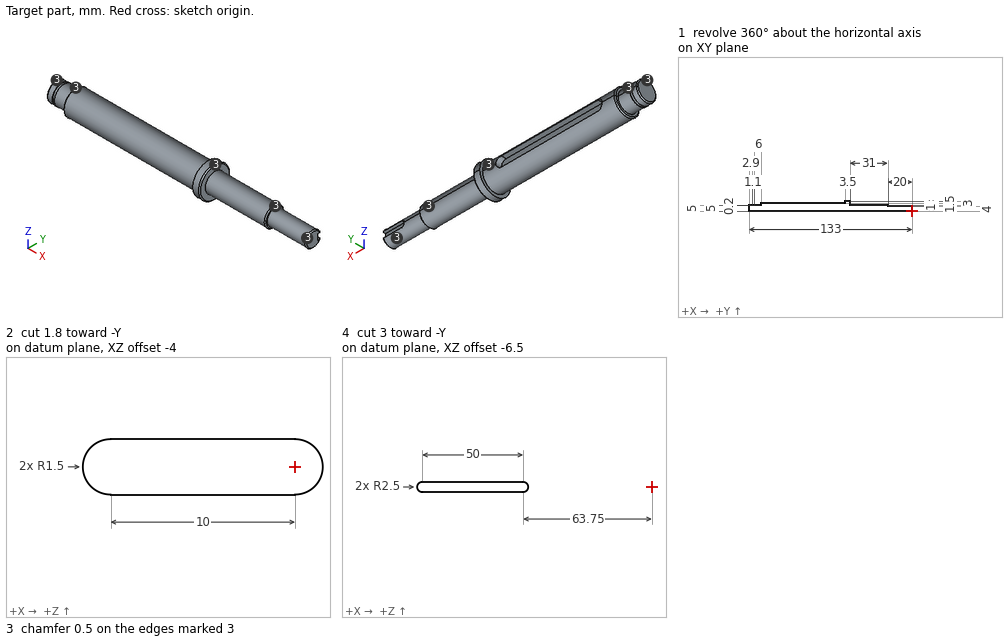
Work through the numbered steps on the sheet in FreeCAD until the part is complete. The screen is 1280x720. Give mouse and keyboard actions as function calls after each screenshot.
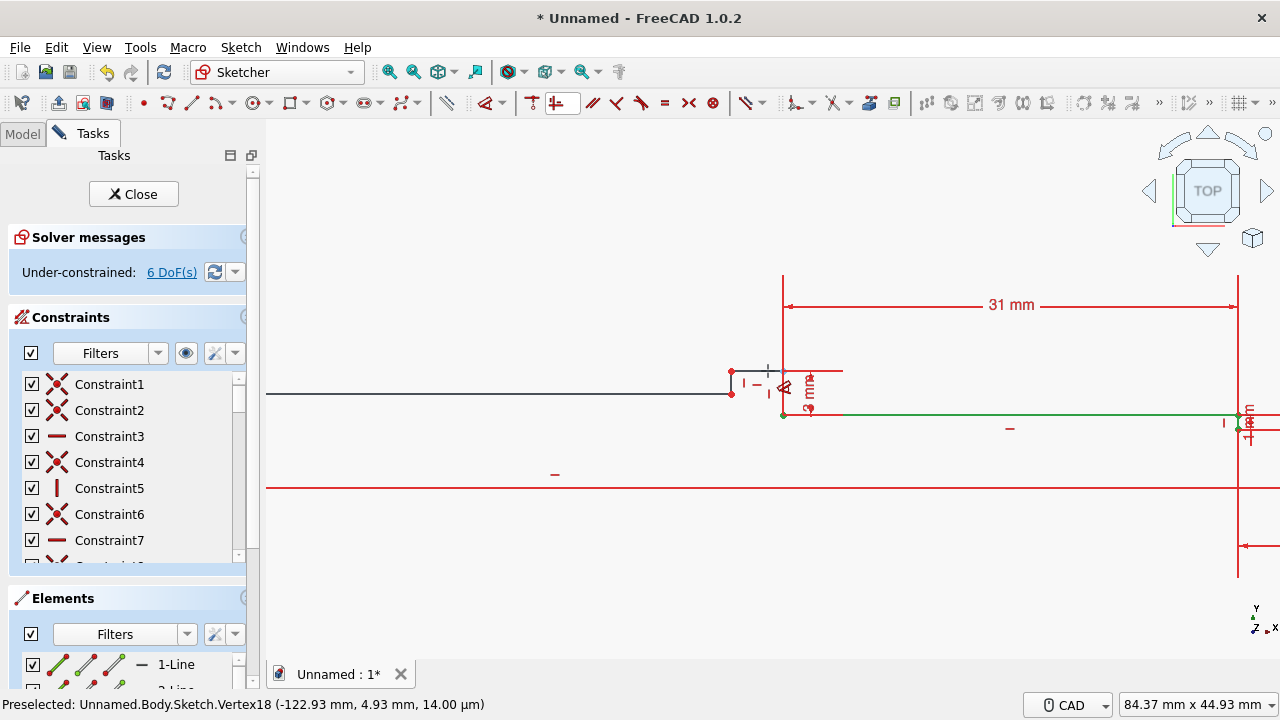
click(768, 371)
click(757, 337)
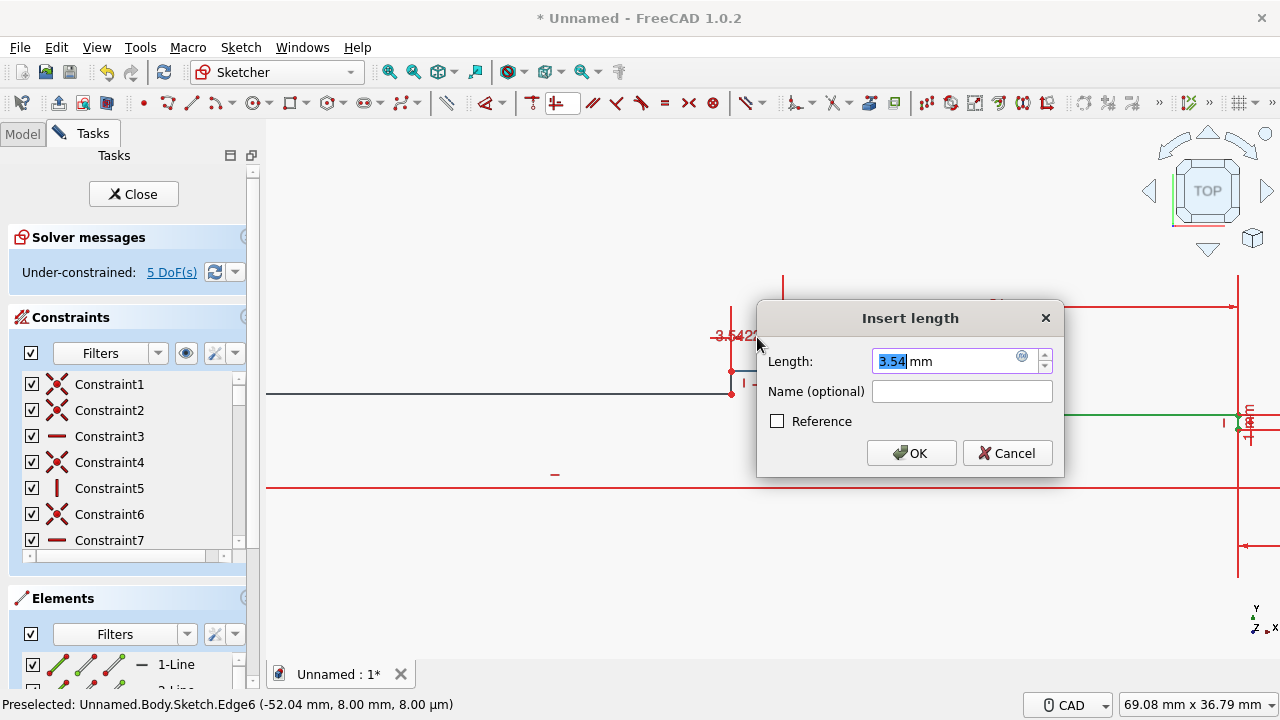
text(3.5)
key(Return)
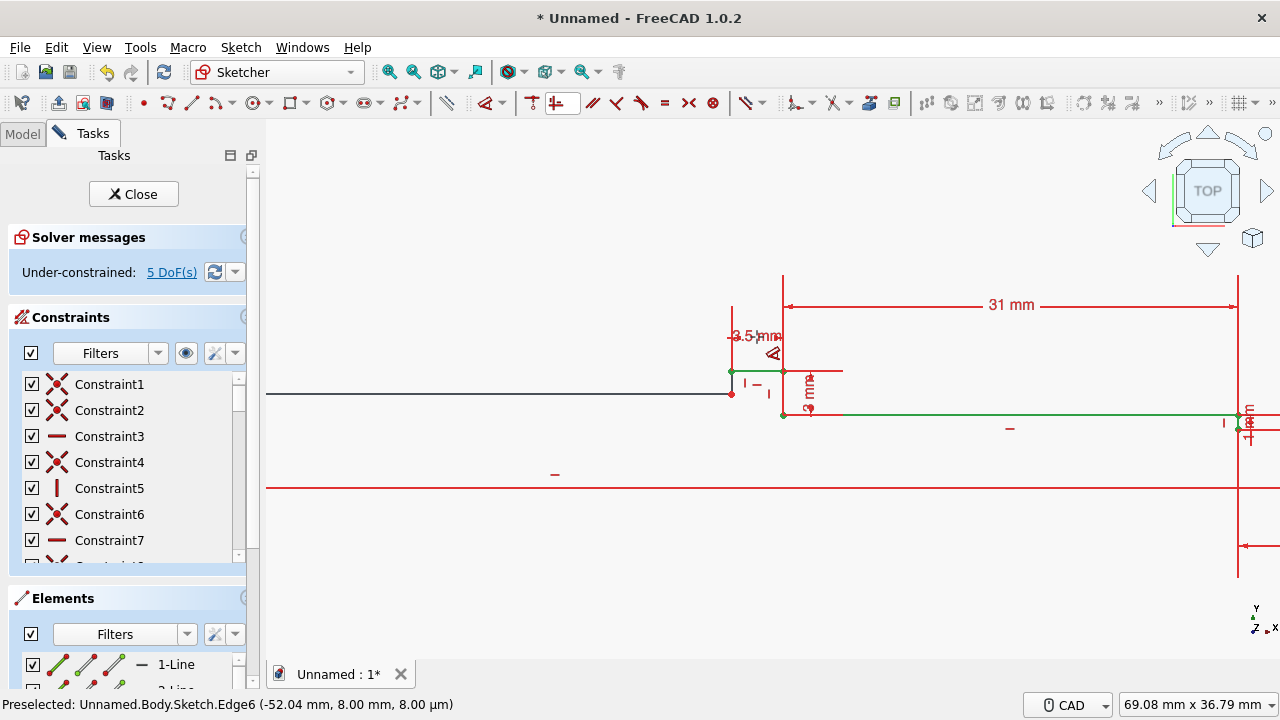
scroll(732, 380, up, 3)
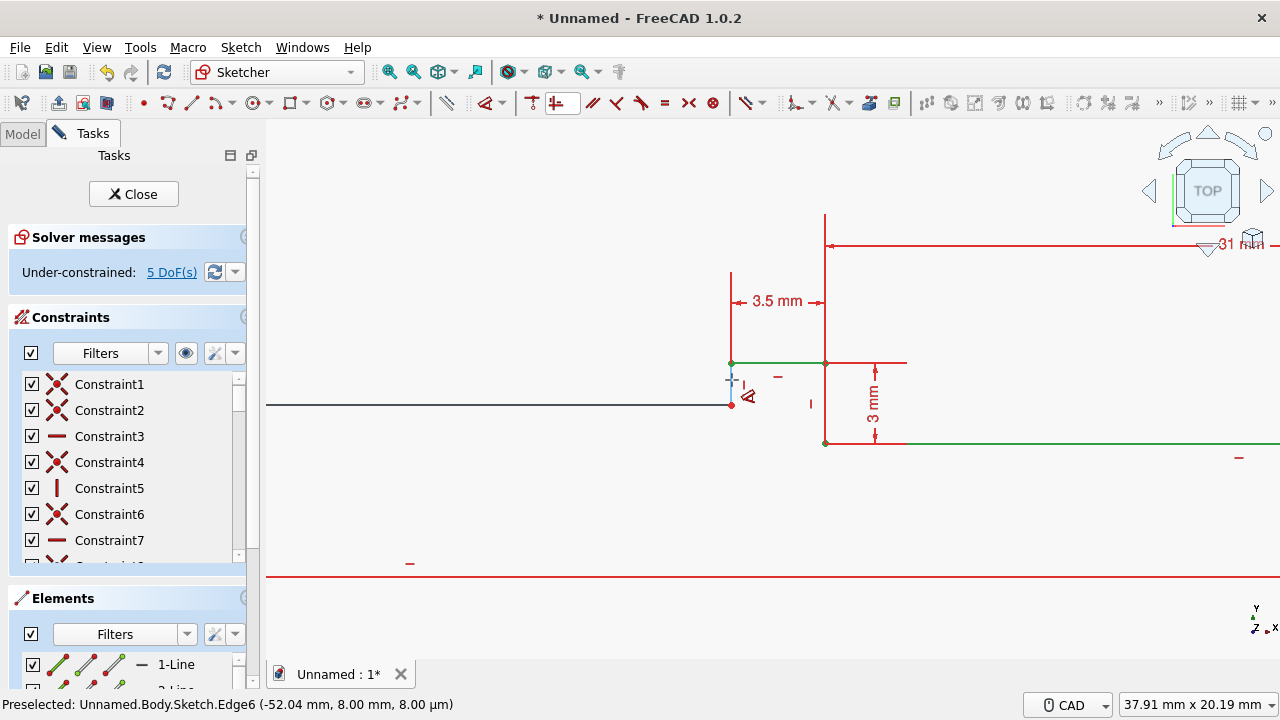
click(731, 380)
click(765, 384)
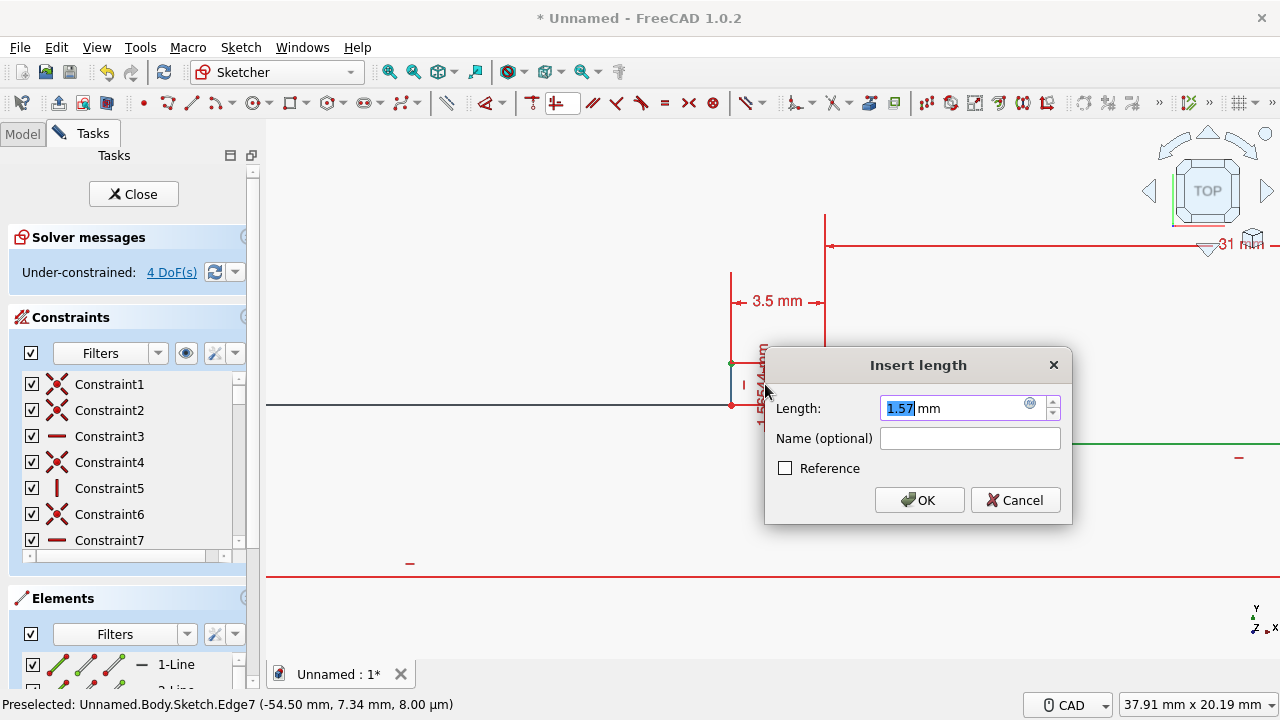
text(1.5)
key(Return)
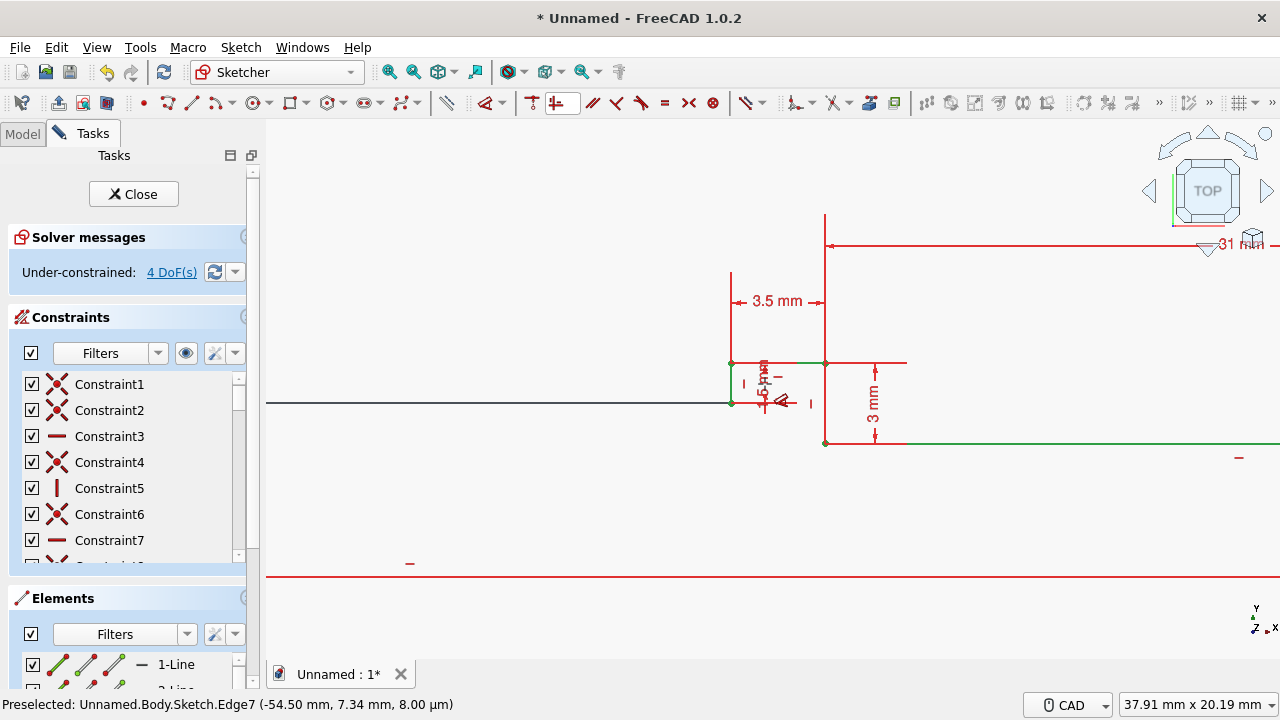
scroll(763, 373, down, 9)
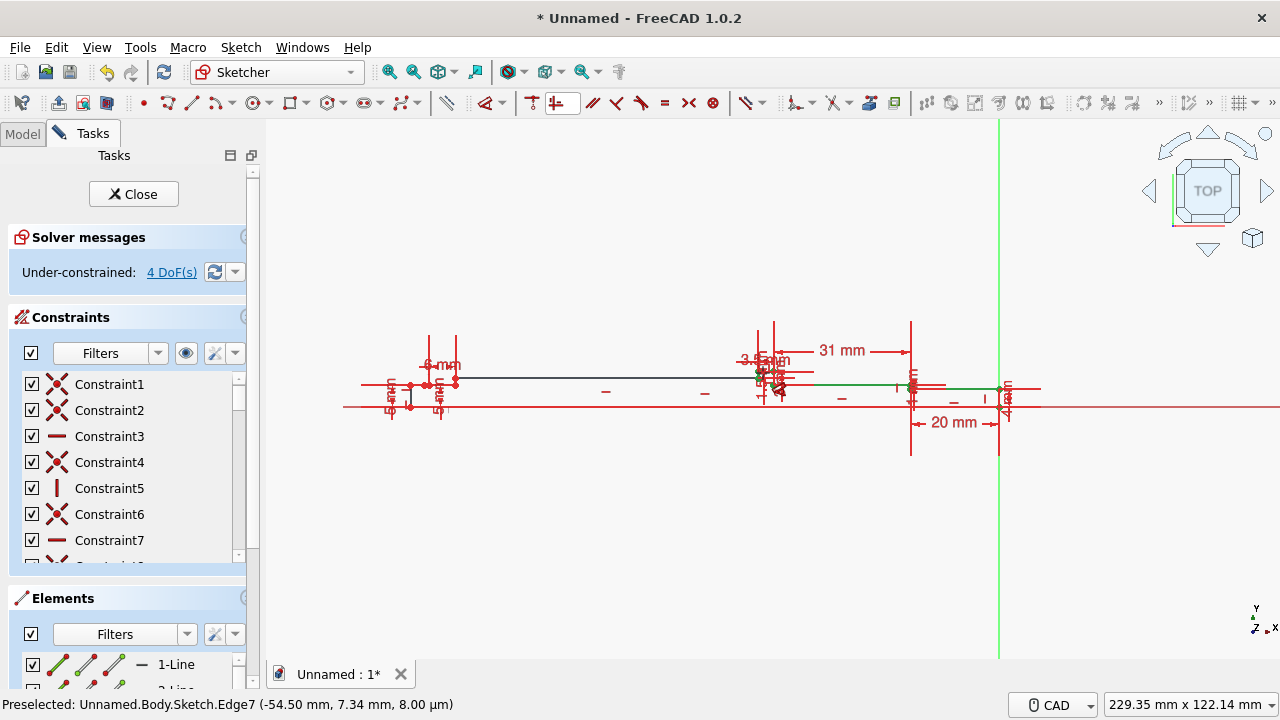
scroll(429, 386, up, 20)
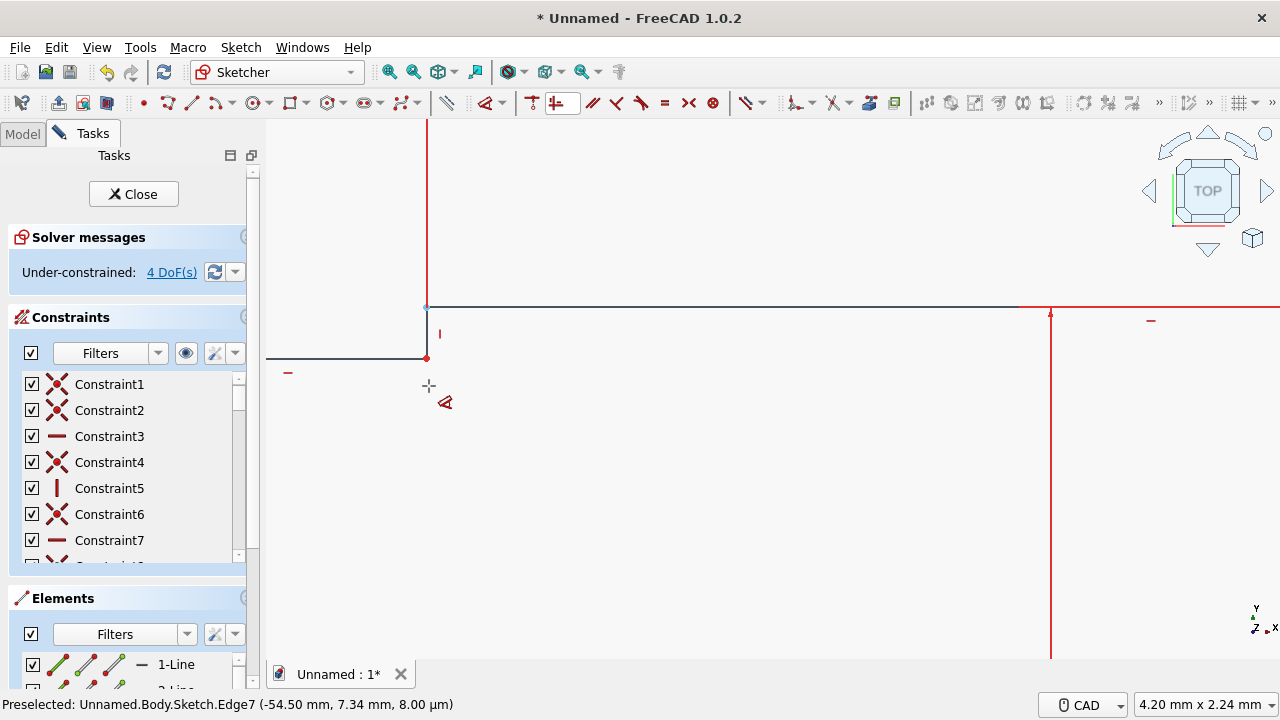
click(427, 333)
click(393, 333)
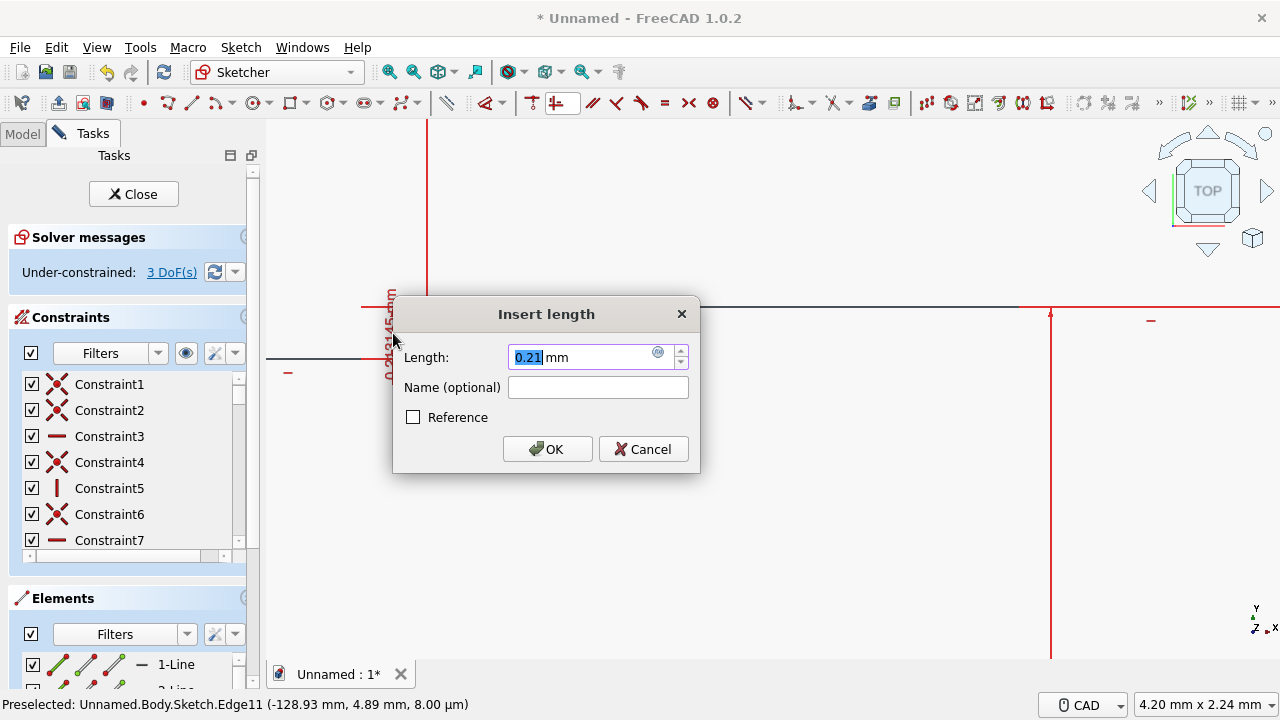
text(0.2)
key(Return)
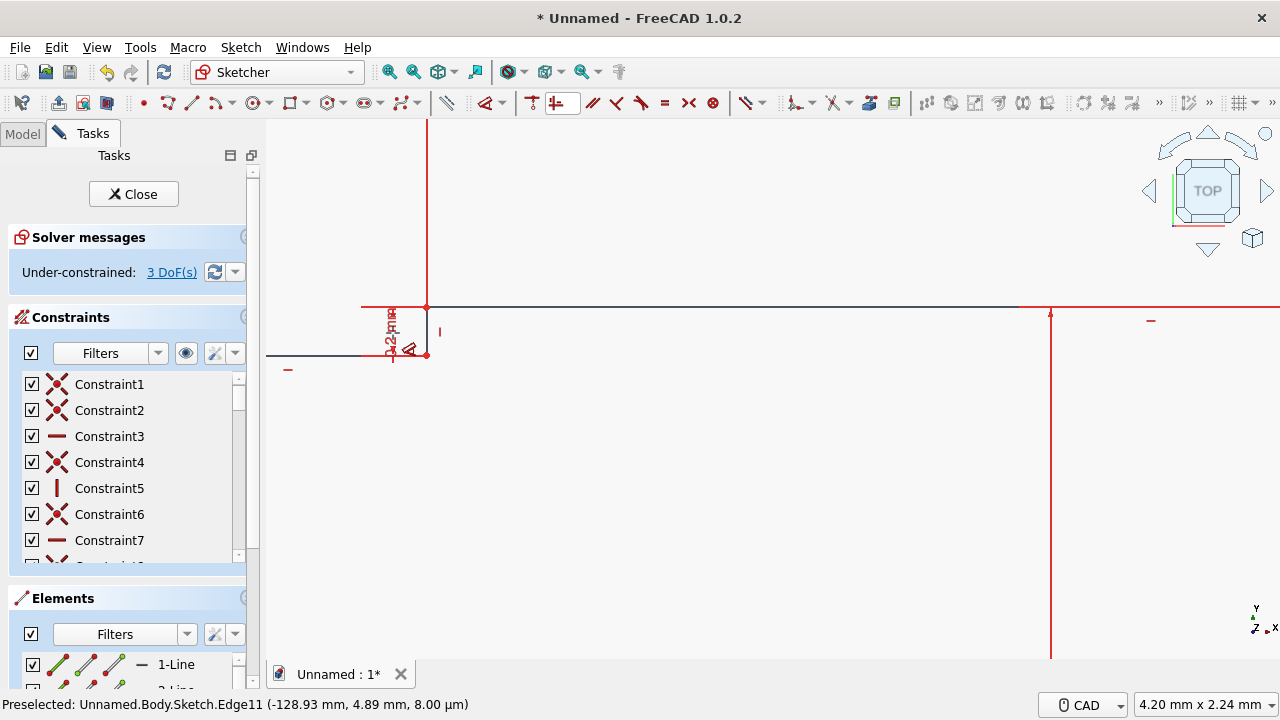
scroll(704, 389, down, 15)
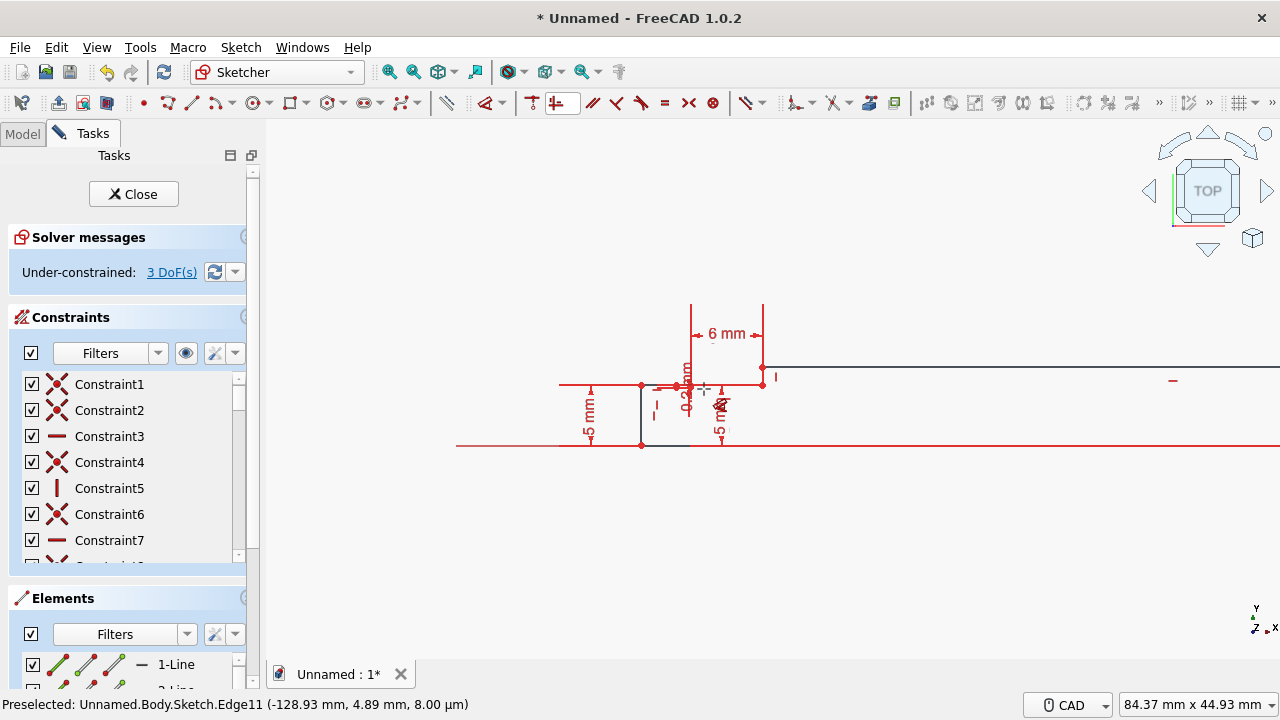
scroll(294, 384, down, 5)